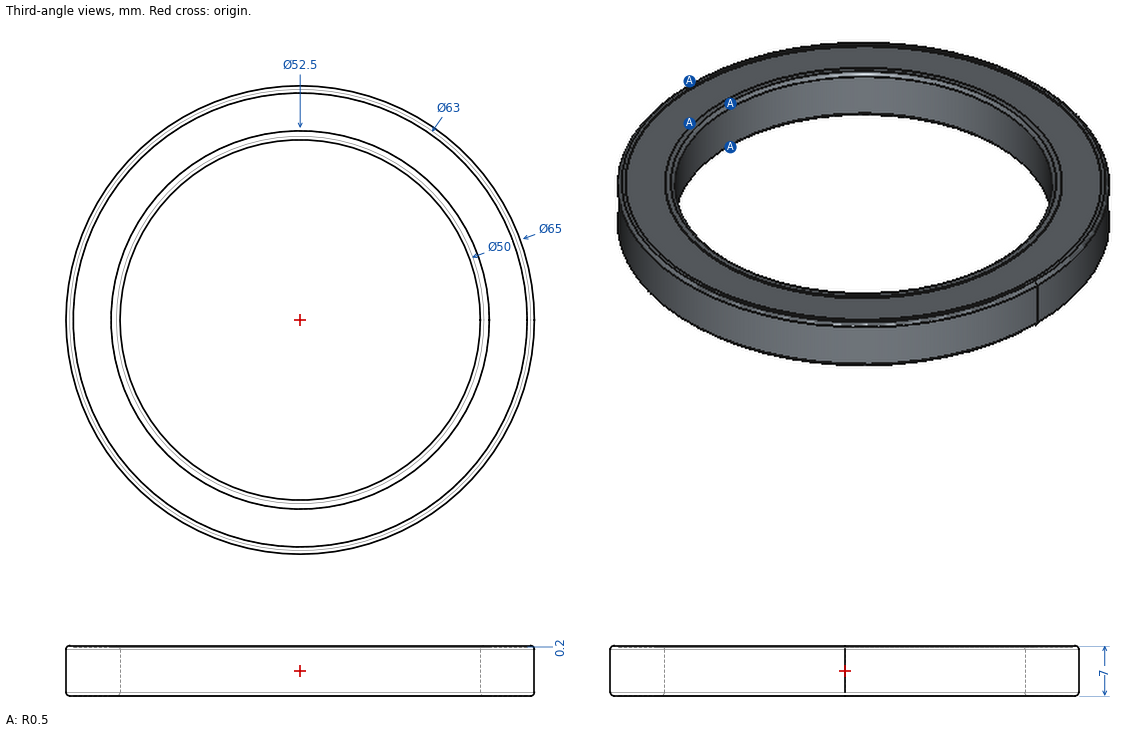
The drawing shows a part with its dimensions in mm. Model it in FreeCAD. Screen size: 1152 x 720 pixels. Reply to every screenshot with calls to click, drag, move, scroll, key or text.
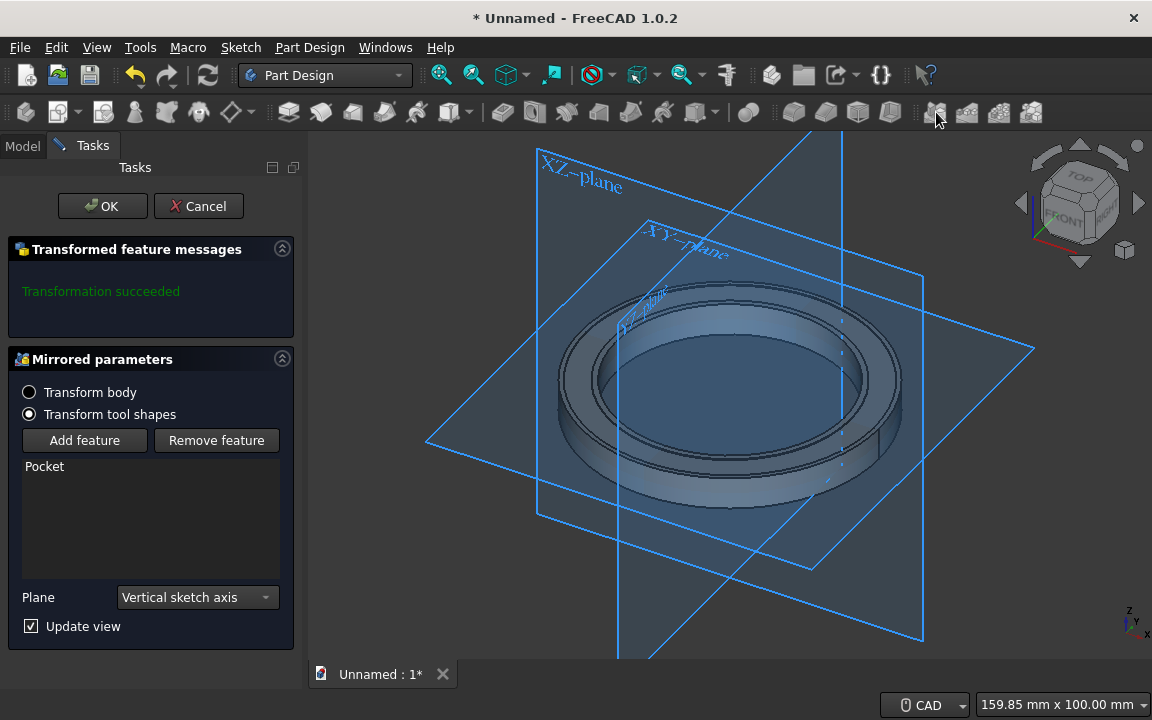
click(198, 598)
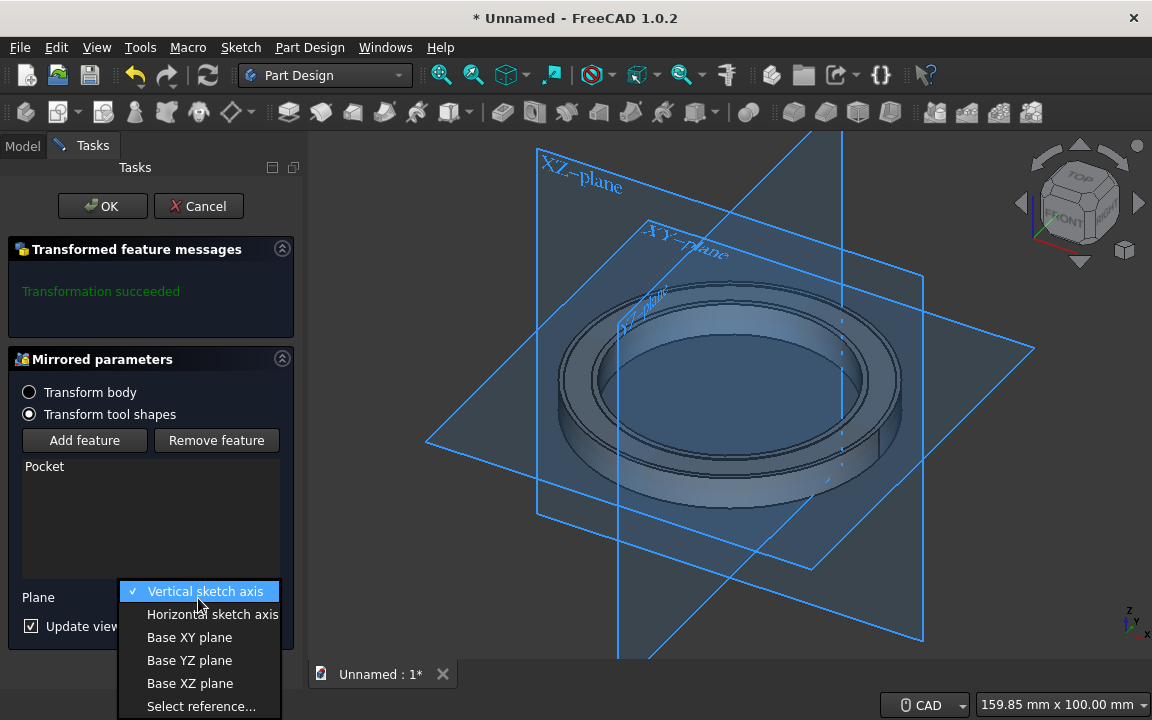
click(198, 638)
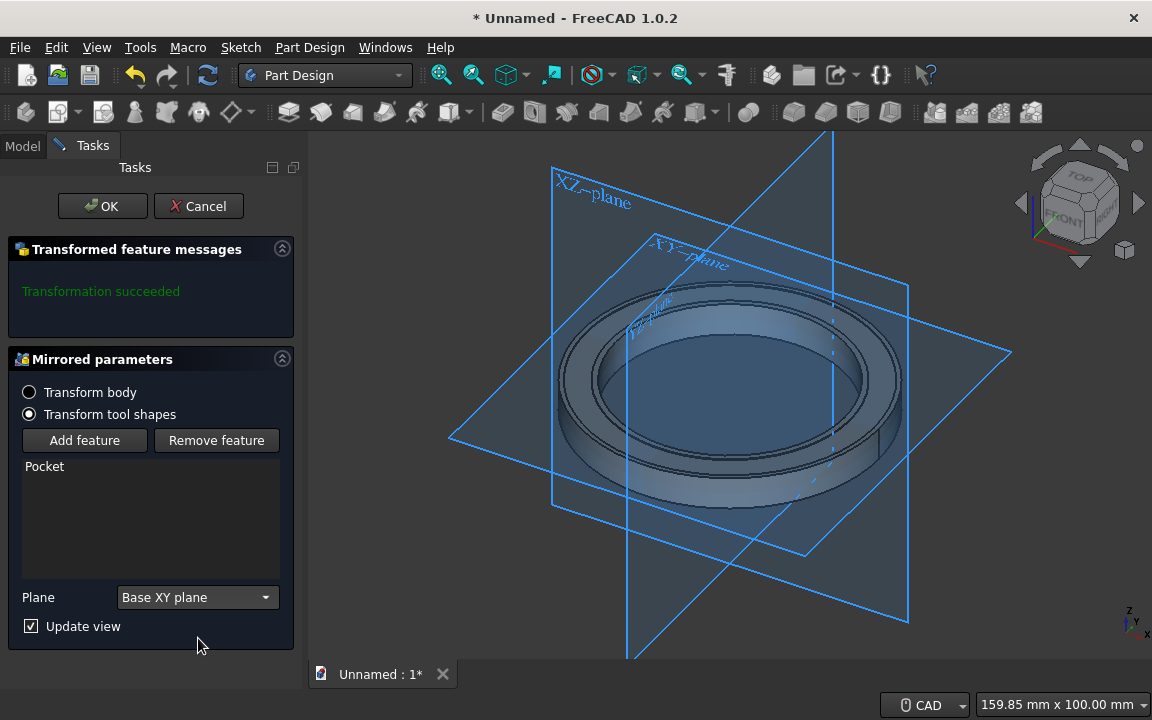
click(103, 206)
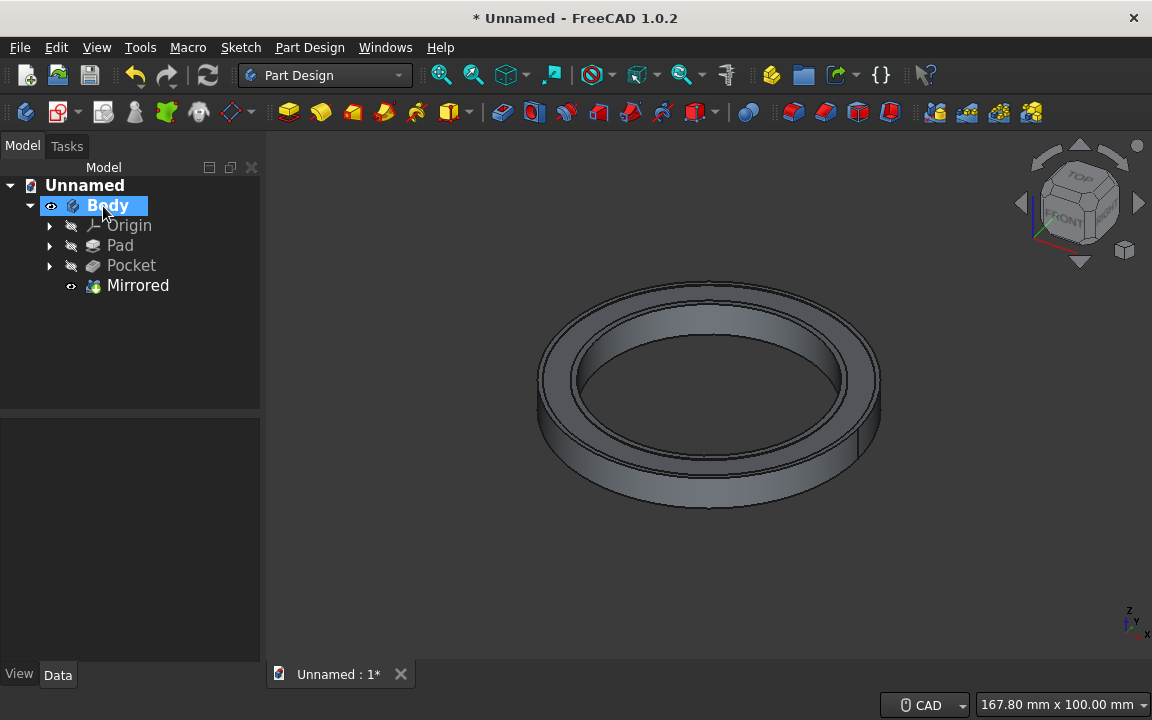
click(538, 389)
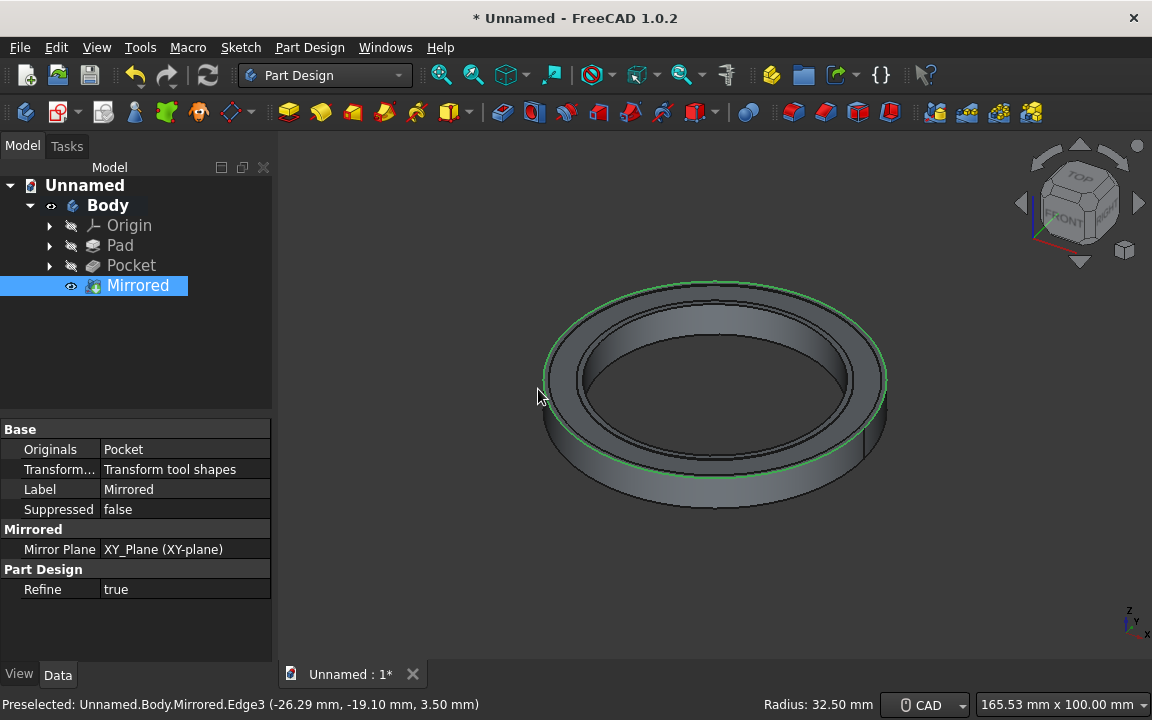
click(601, 341, ctrl)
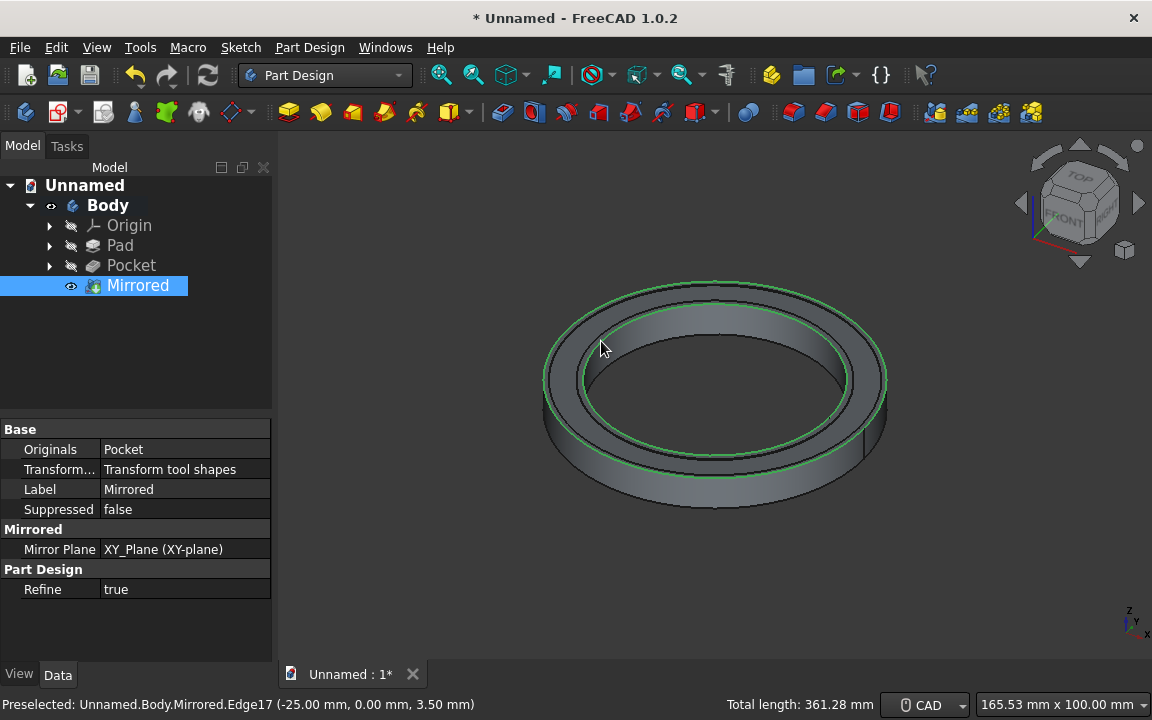
key(0)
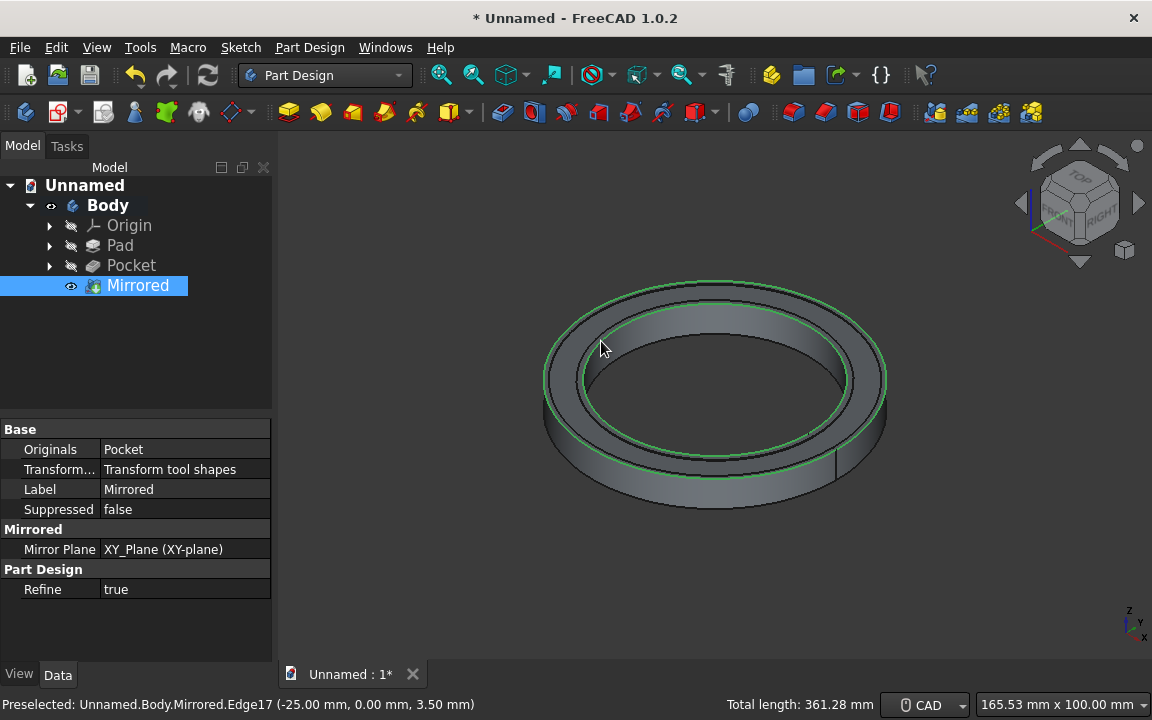
key(2)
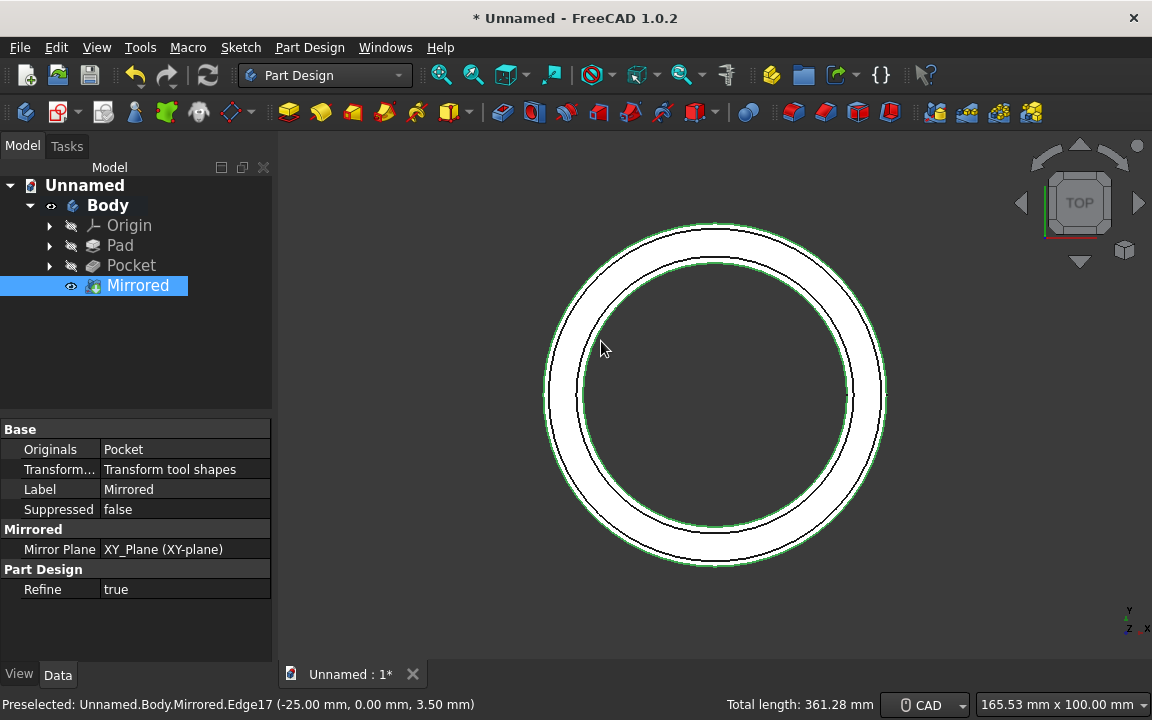
key(1)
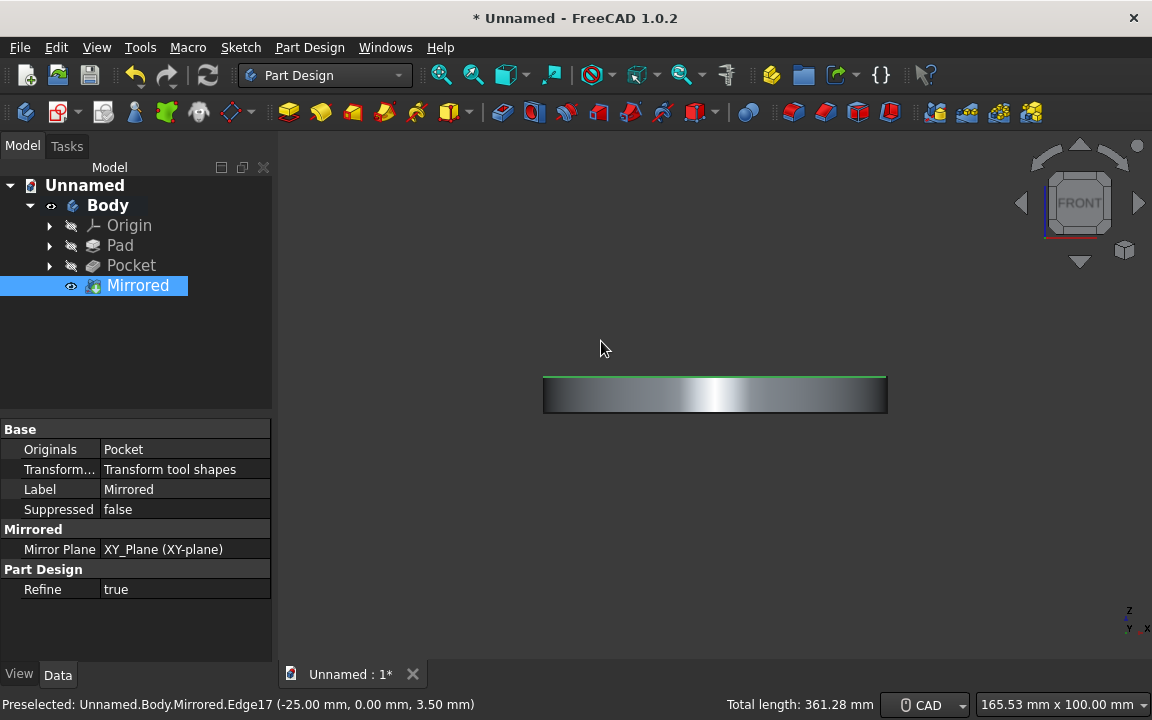
click(442, 76)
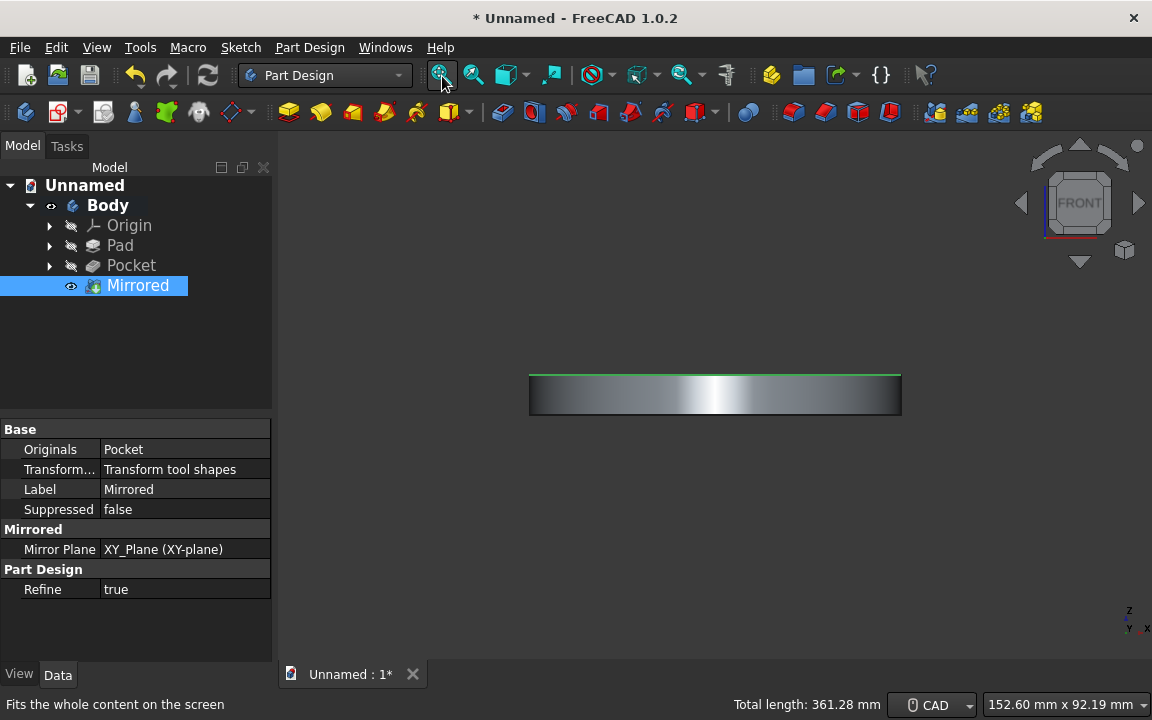
click(564, 414, ctrl)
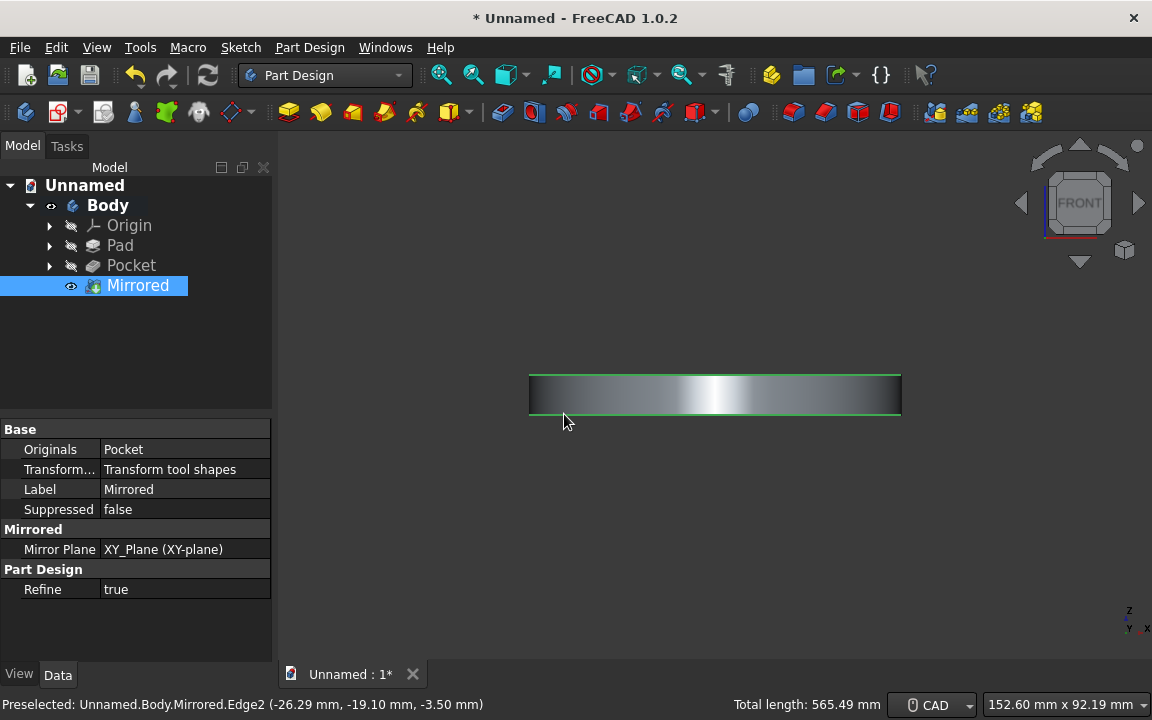
key(3)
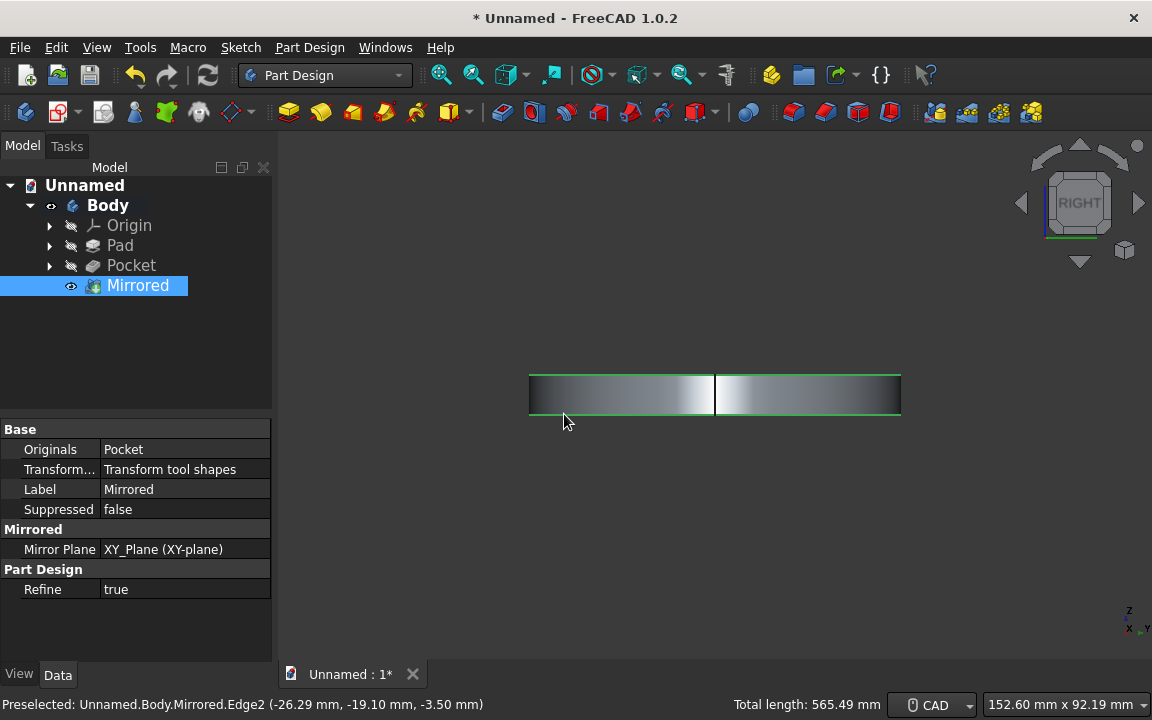
key(v)
key(f)